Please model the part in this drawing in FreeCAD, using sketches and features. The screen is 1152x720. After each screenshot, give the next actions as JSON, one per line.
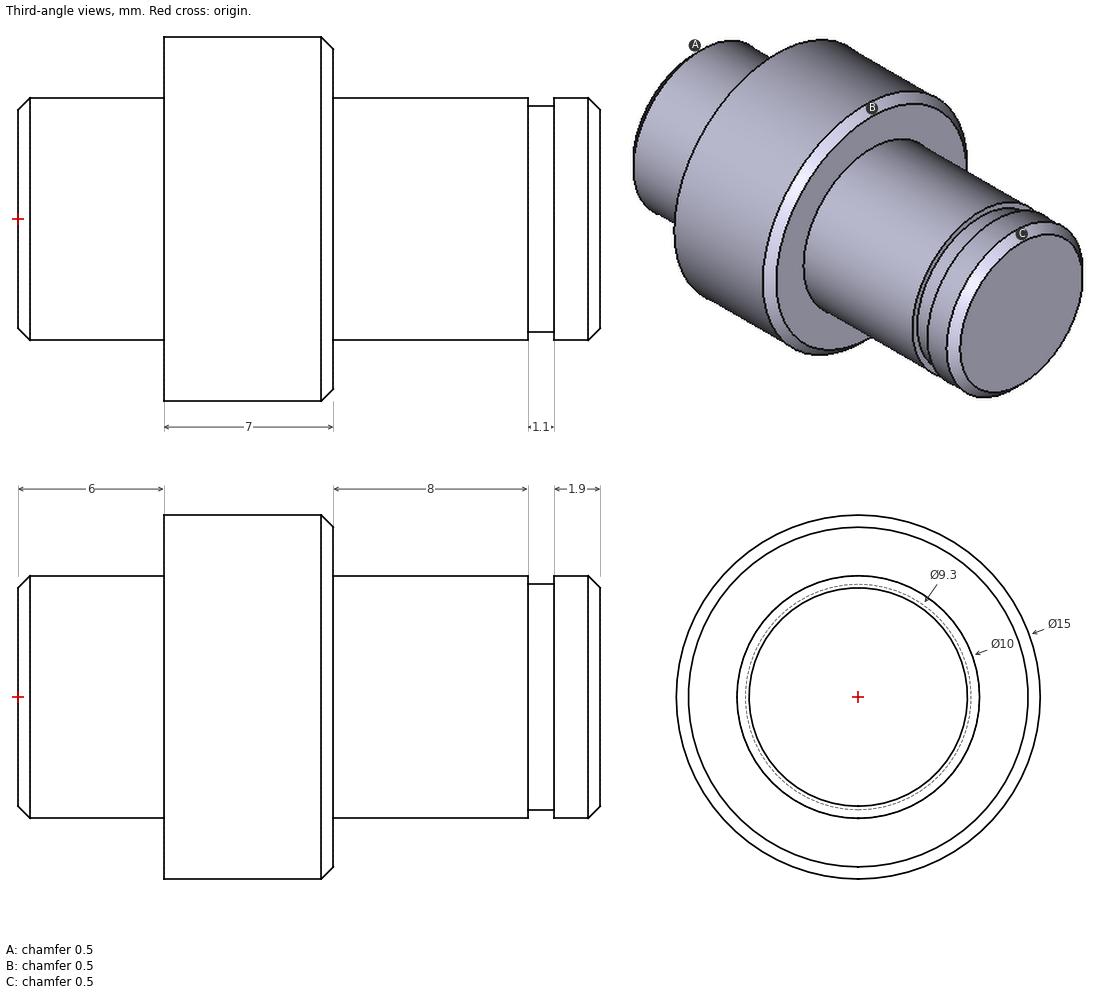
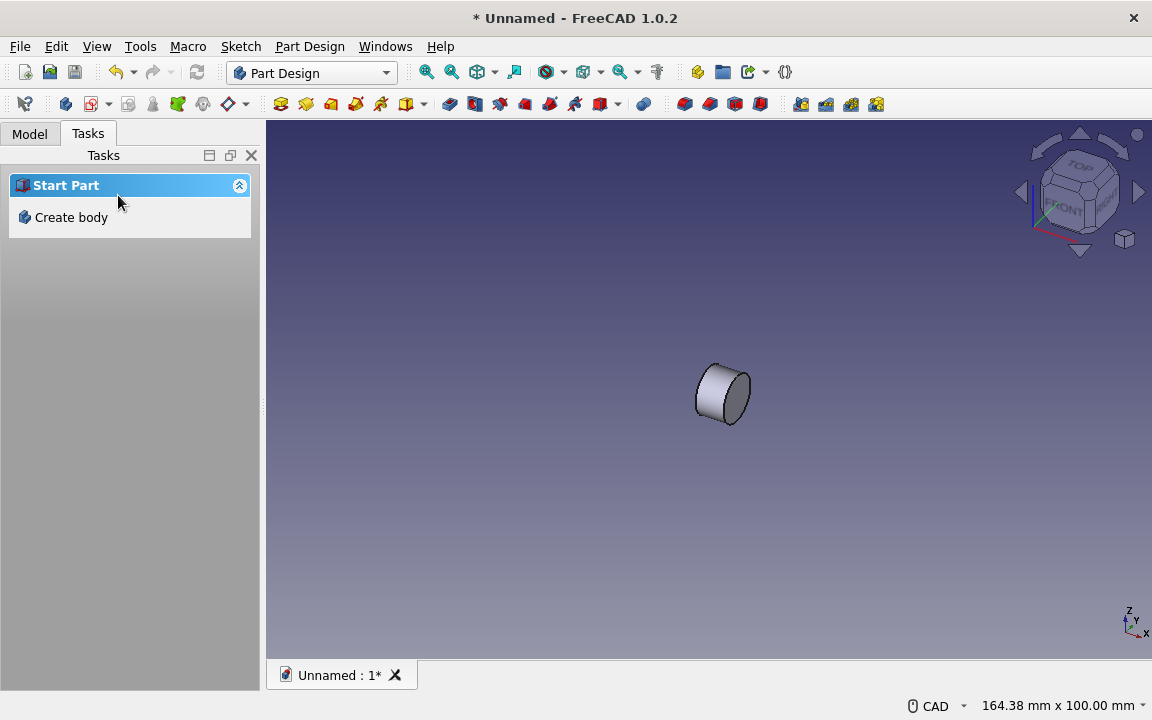
{"action": "left_click", "coordinate": [427, 72]}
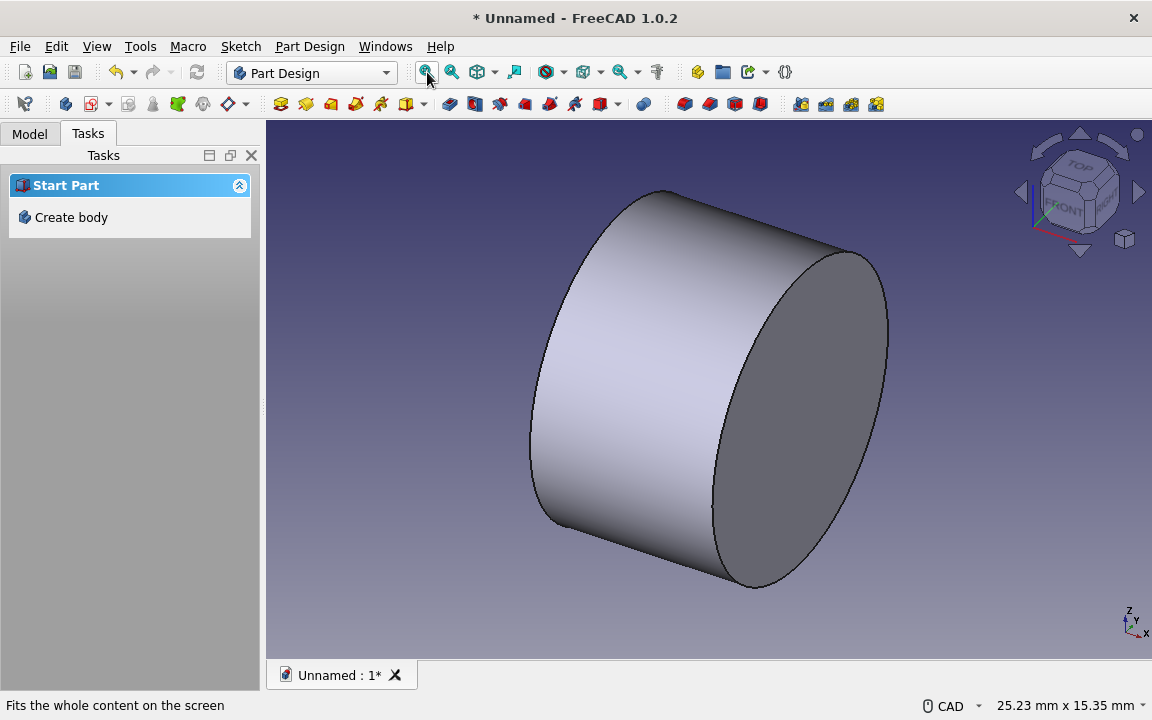
{"action": "key", "text": "0"}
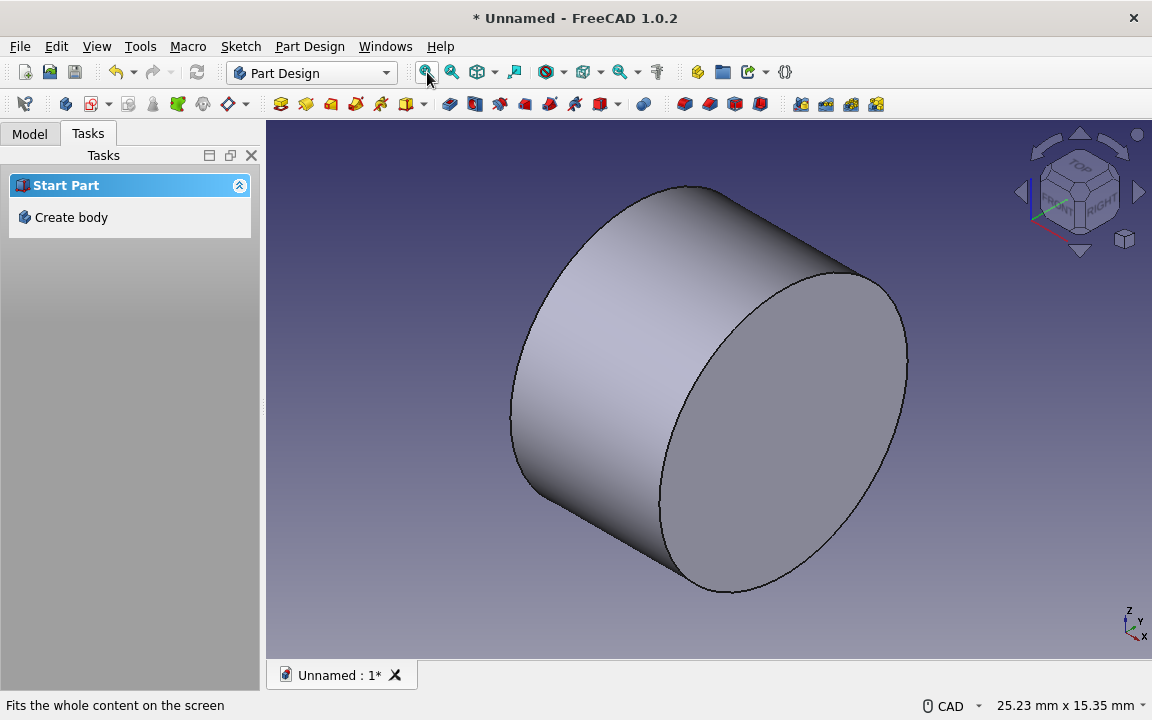
{"action": "key", "text": "2"}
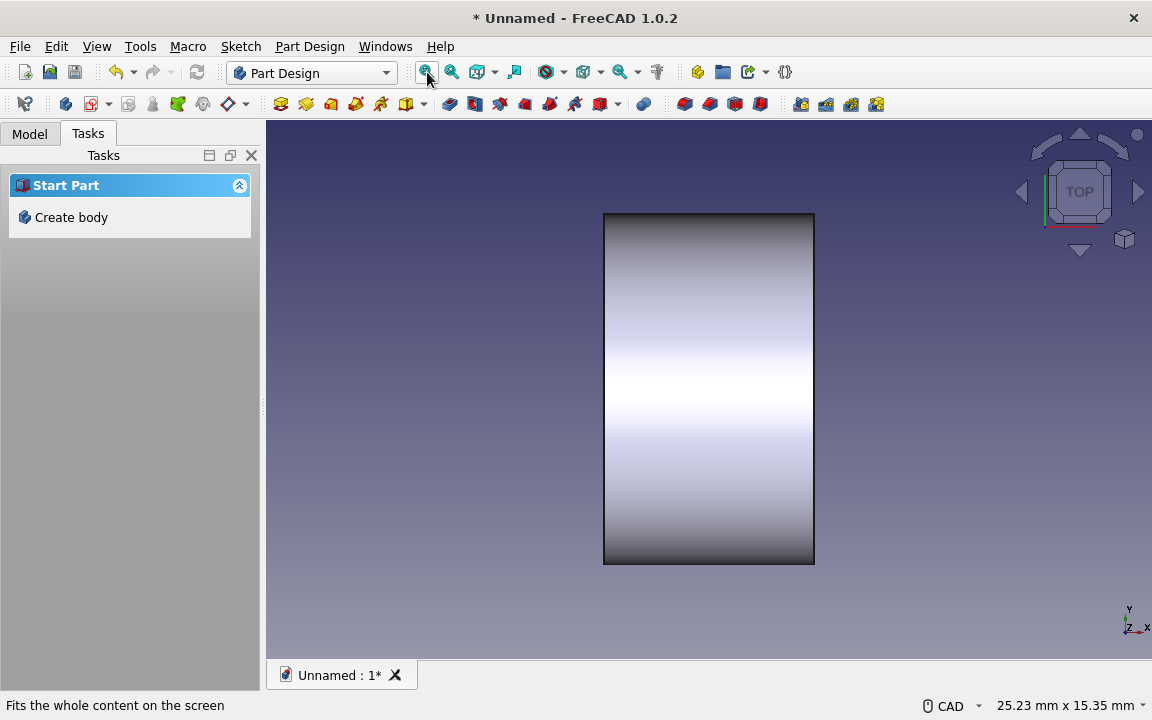
{"action": "left_click", "coordinate": [604, 531]}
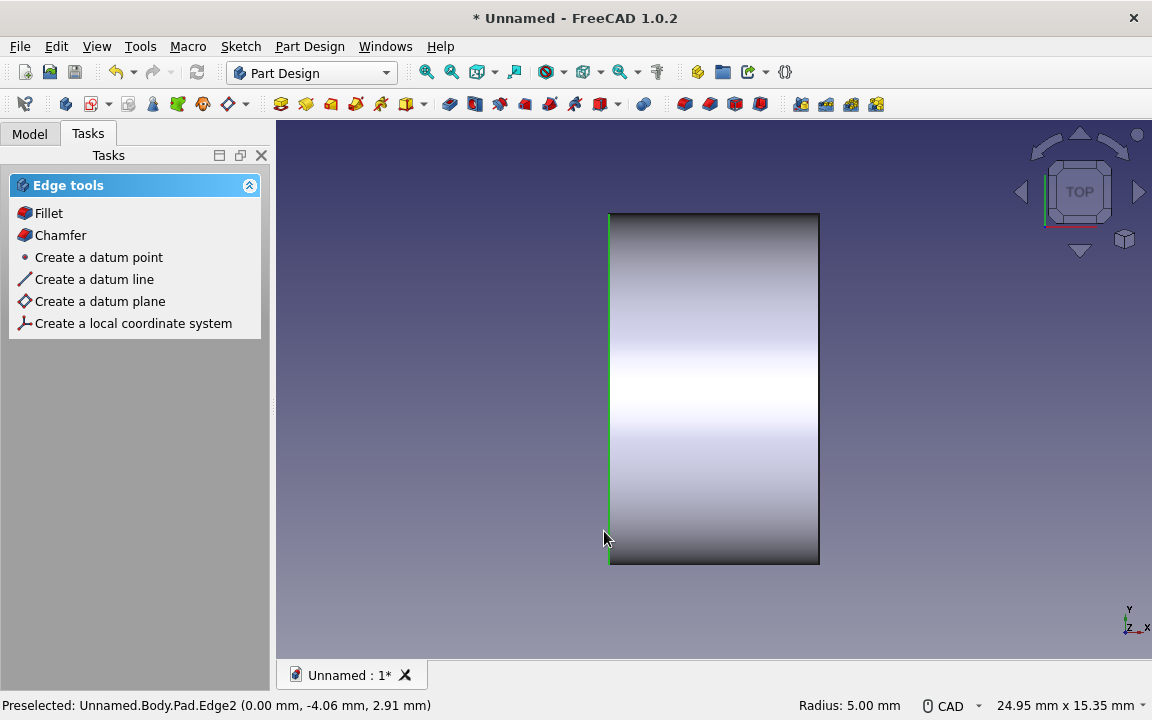
{"action": "left_click", "coordinate": [710, 104]}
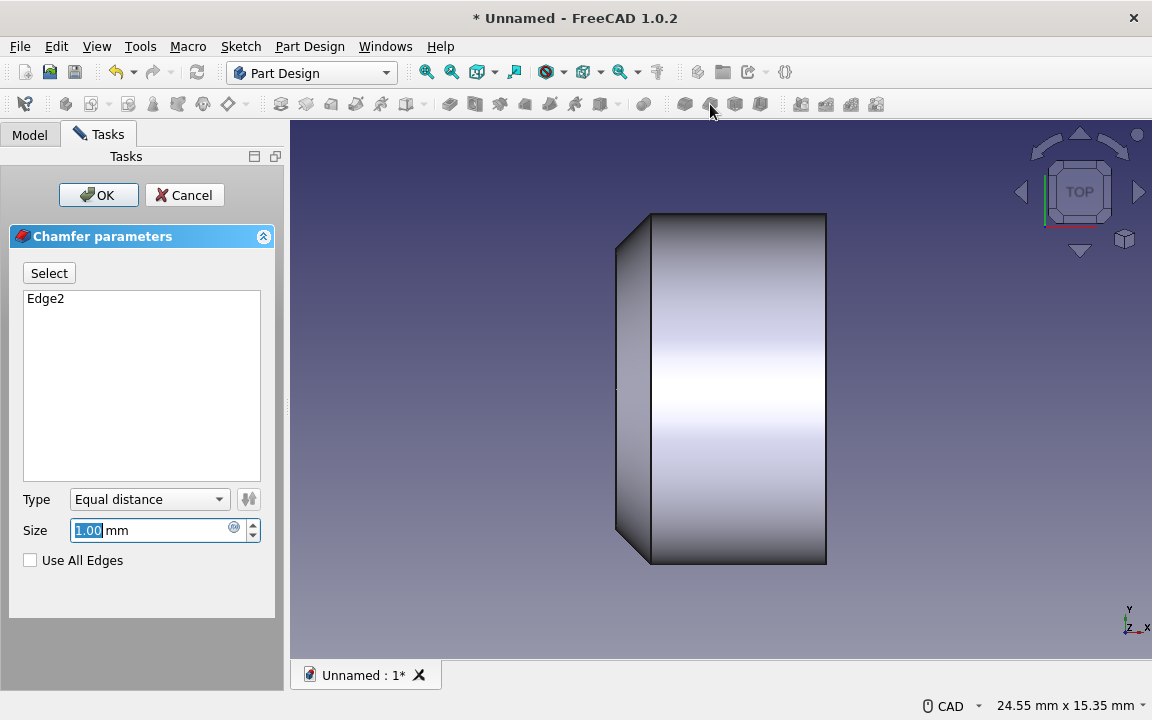
{"action": "type", "text": "0.5"}
{"action": "key", "text": "Tab"}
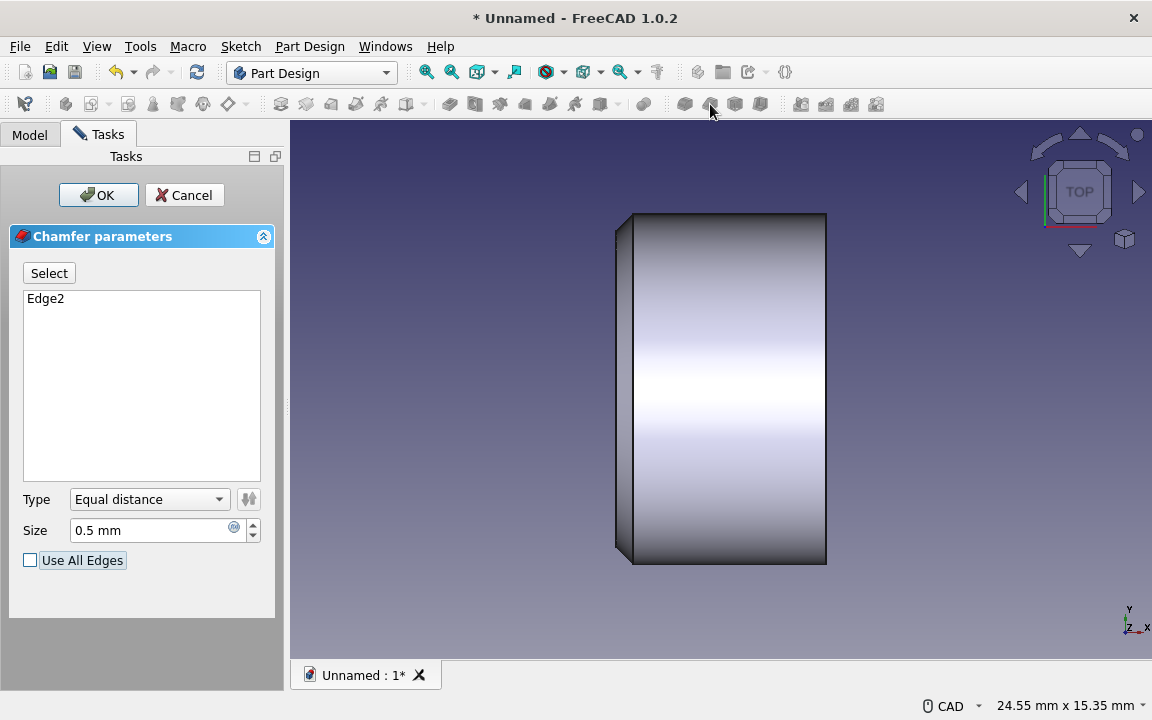
{"action": "left_click", "coordinate": [99, 195]}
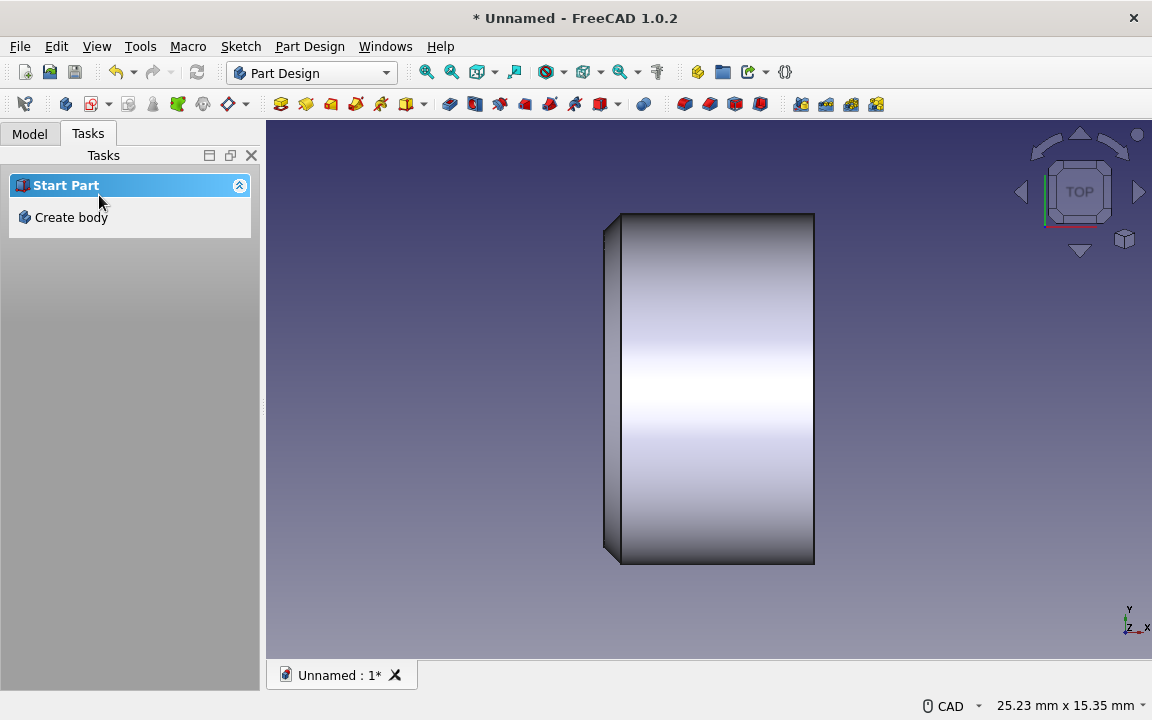
{"action": "key", "text": "0"}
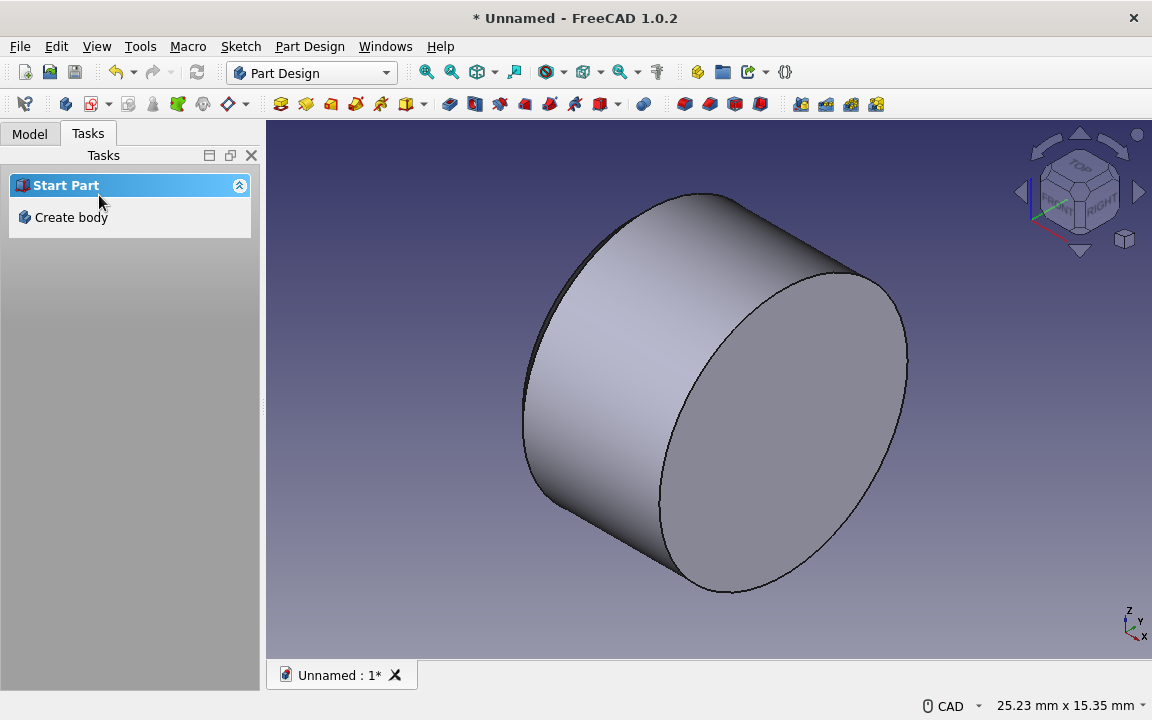
{"action": "left_click", "coordinate": [783, 432]}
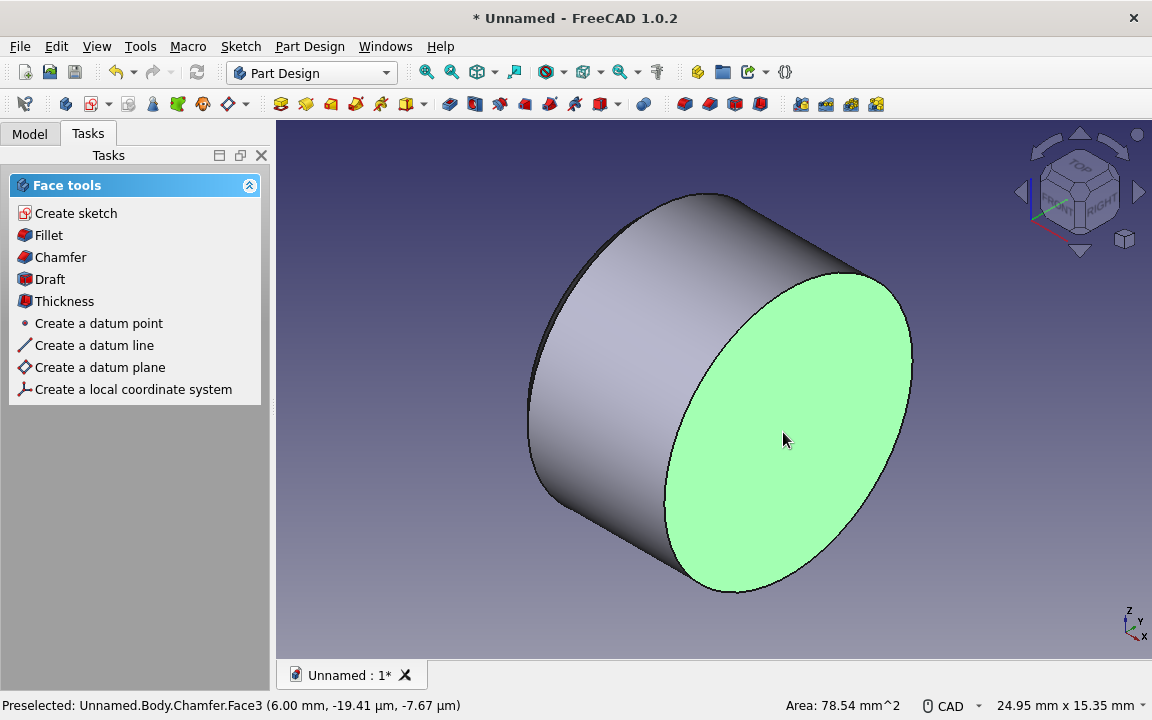
{"action": "left_click", "coordinate": [90, 104]}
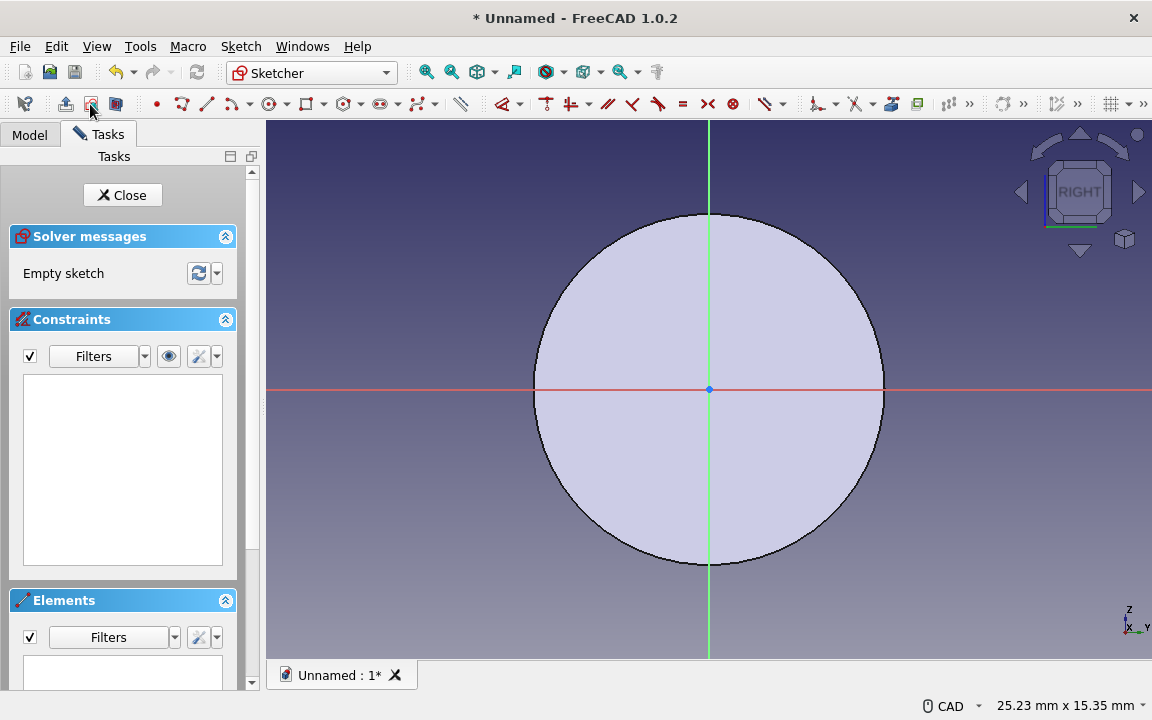
{"action": "scroll", "coordinate": [501, 390], "scroll_direction": "down", "scroll_amount": 2}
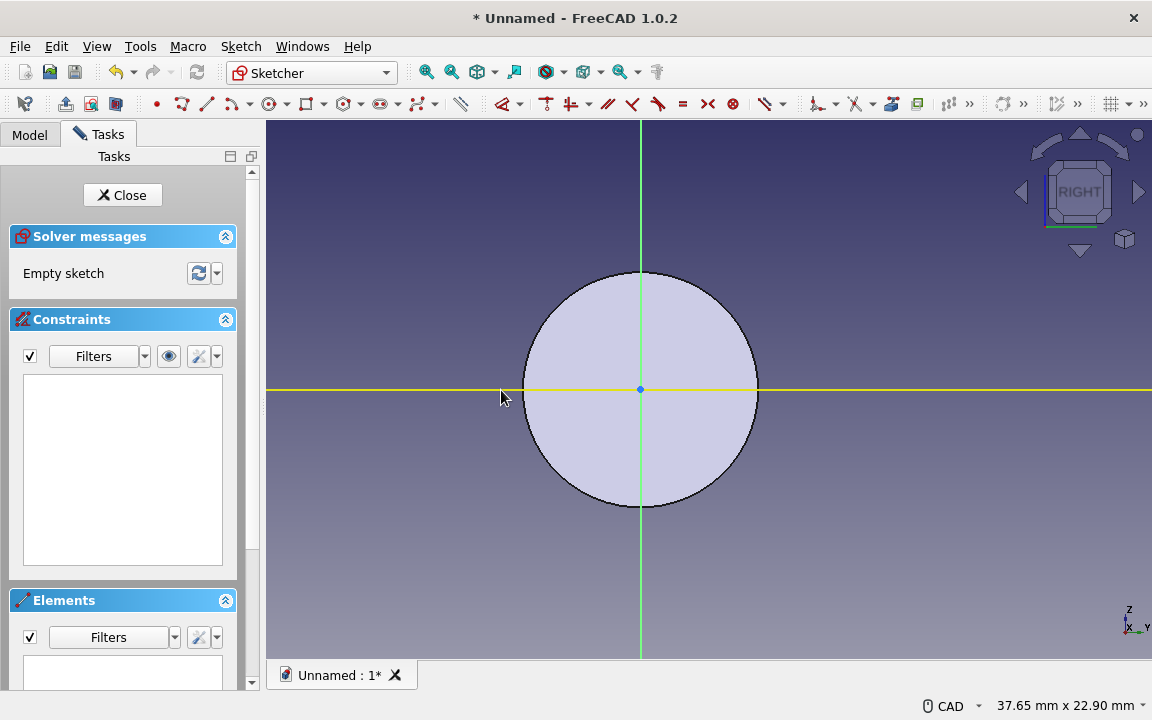
{"action": "key", "text": "g c"}